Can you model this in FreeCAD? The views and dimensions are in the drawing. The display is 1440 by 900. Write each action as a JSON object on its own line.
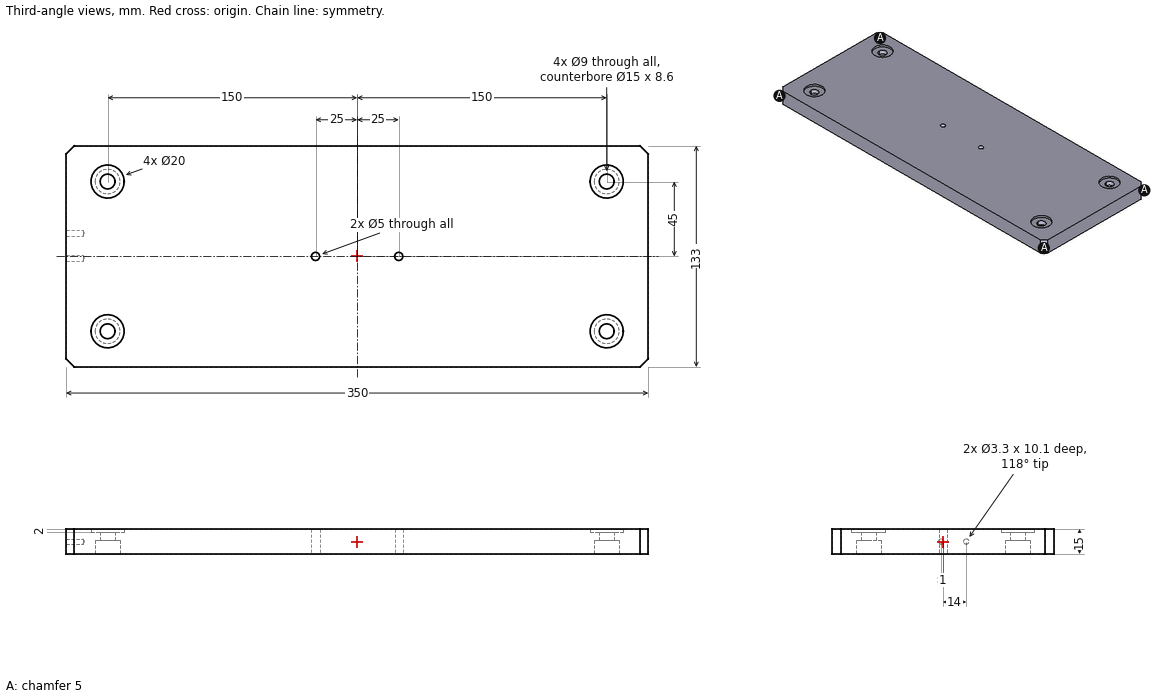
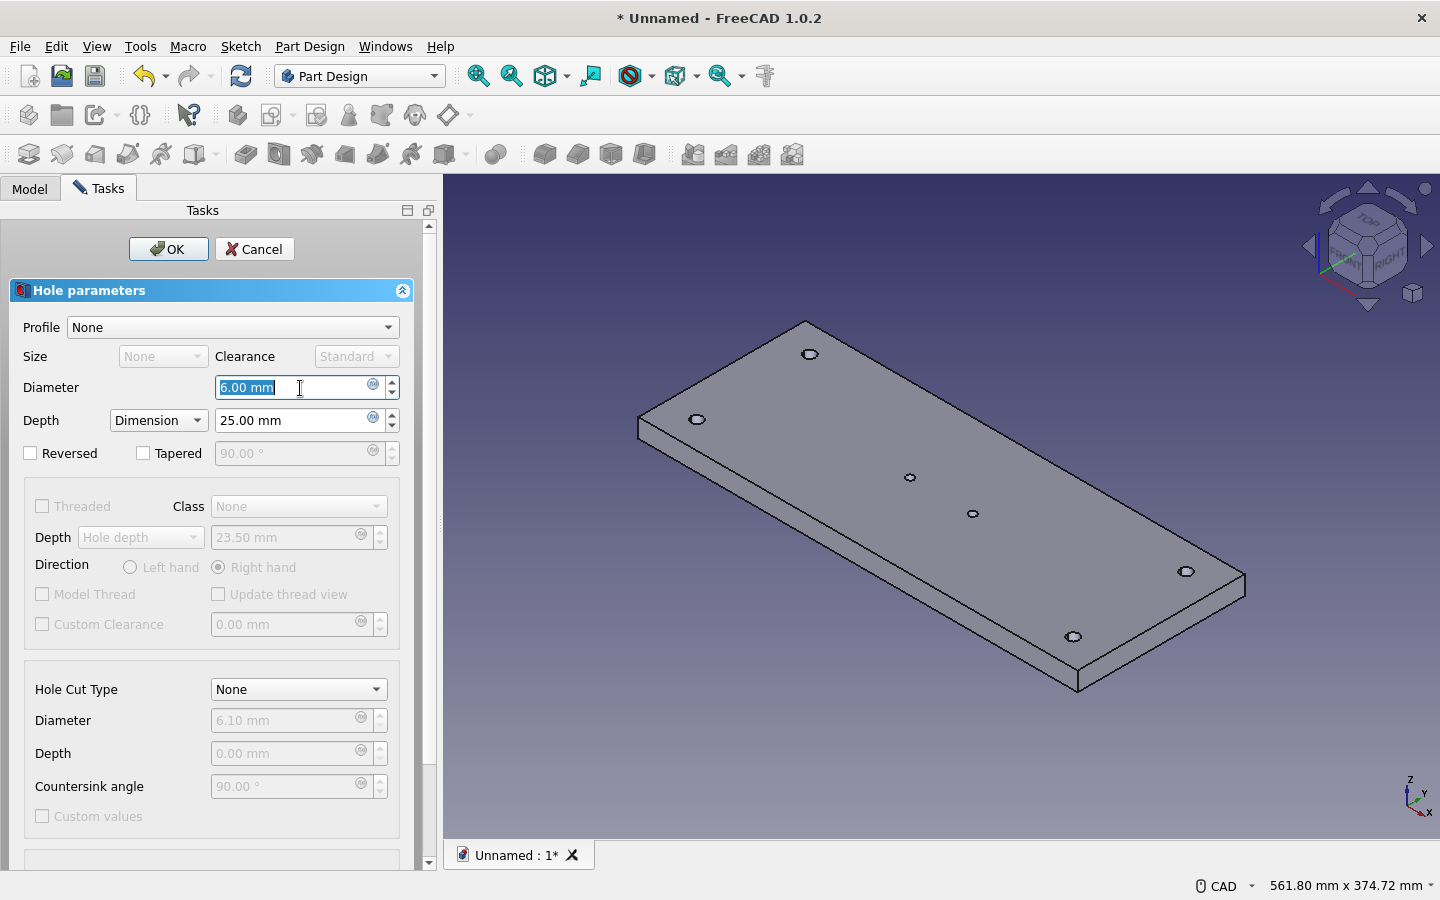
{"action": "type", "text": "5"}
{"action": "key", "text": "Tab"}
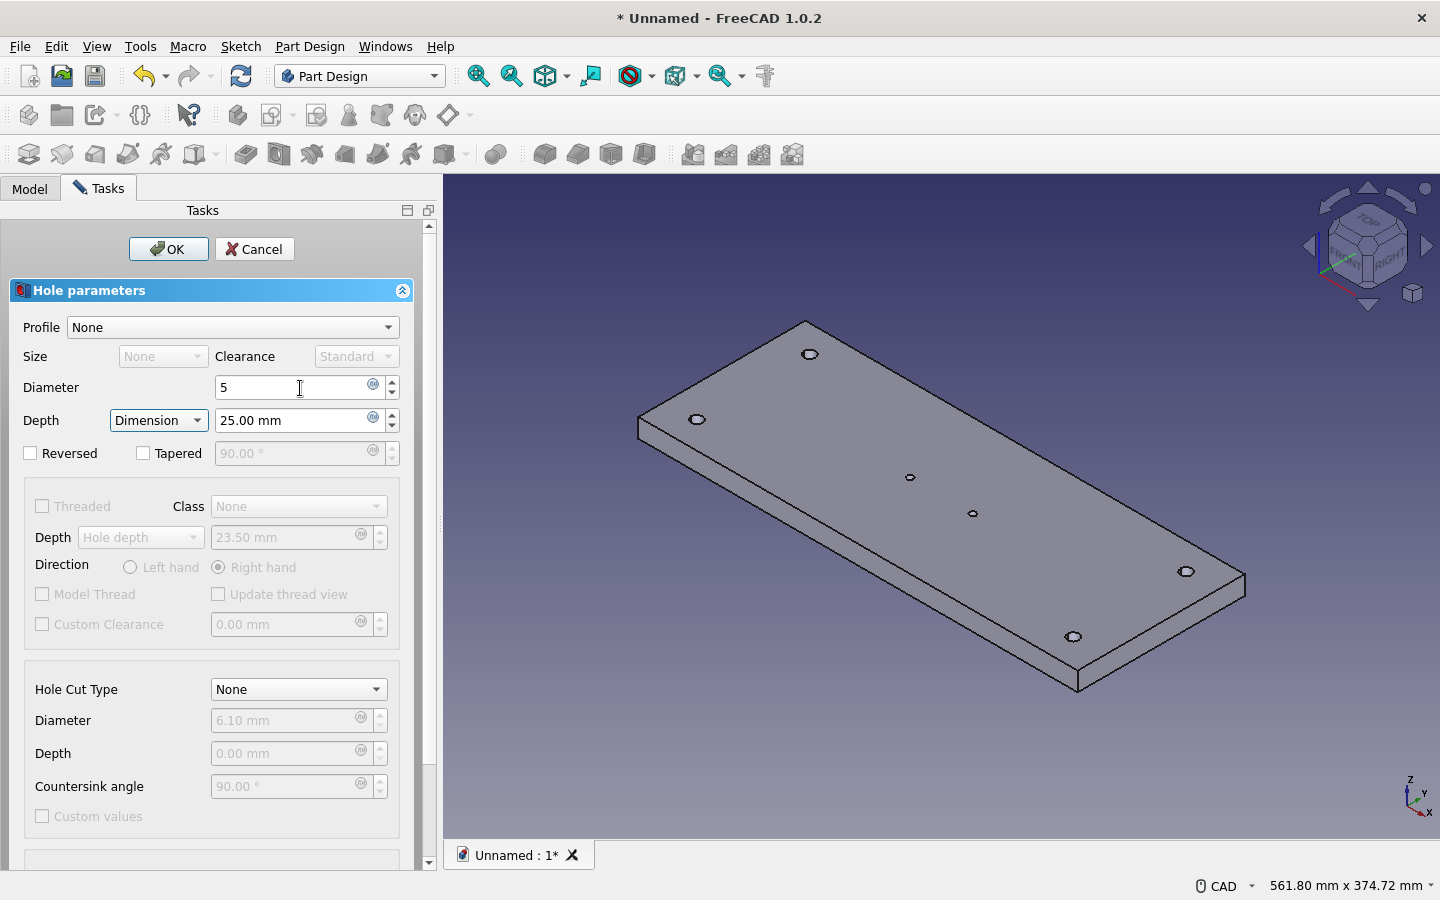
{"action": "left_click", "coordinate": [160, 420]}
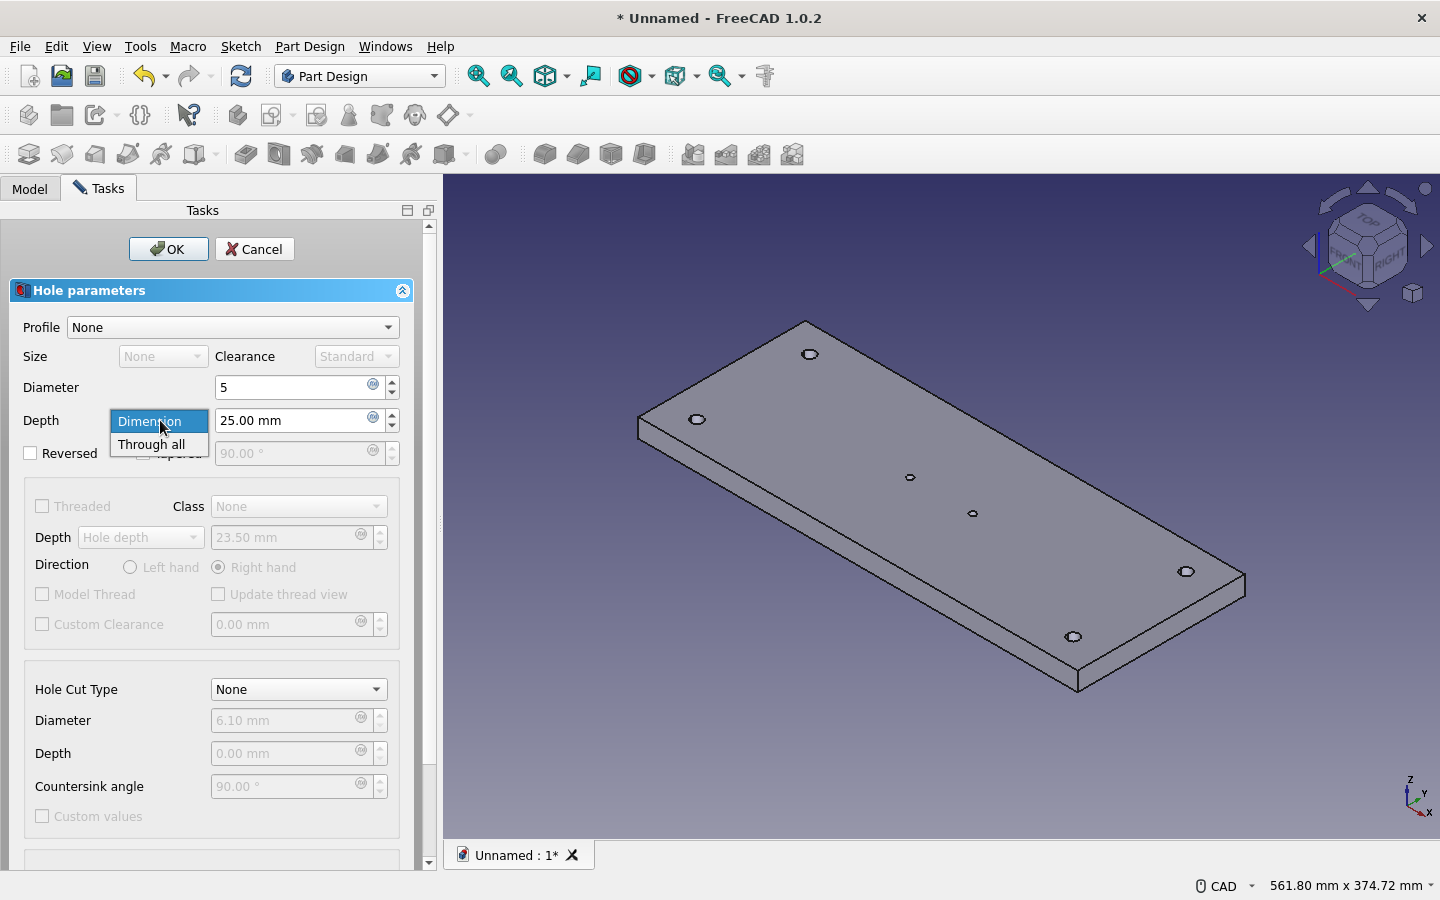
{"action": "left_click", "coordinate": [158, 444]}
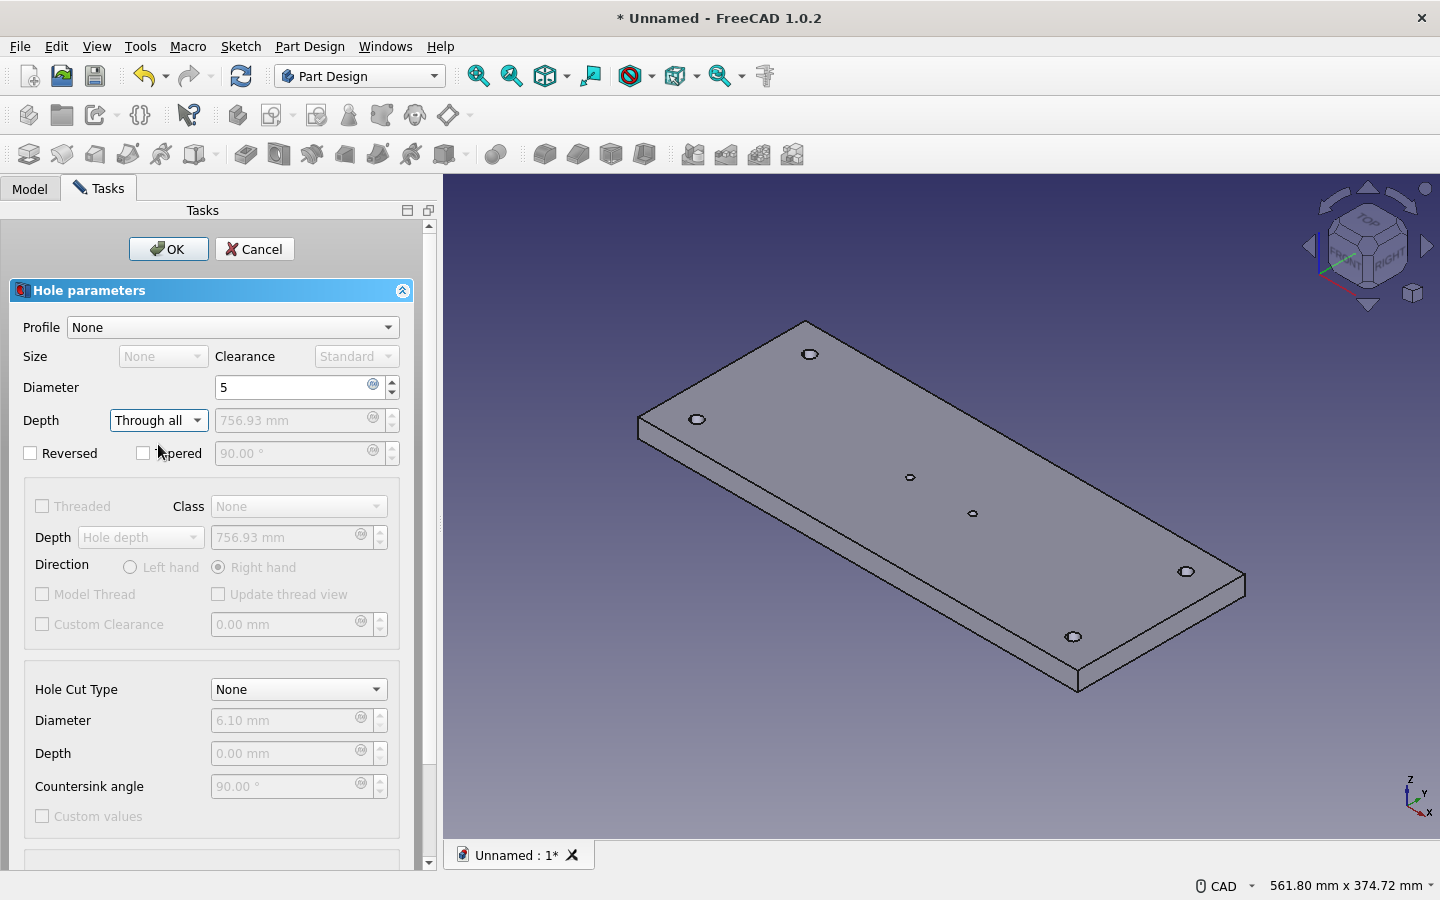
{"action": "left_click", "coordinate": [169, 249]}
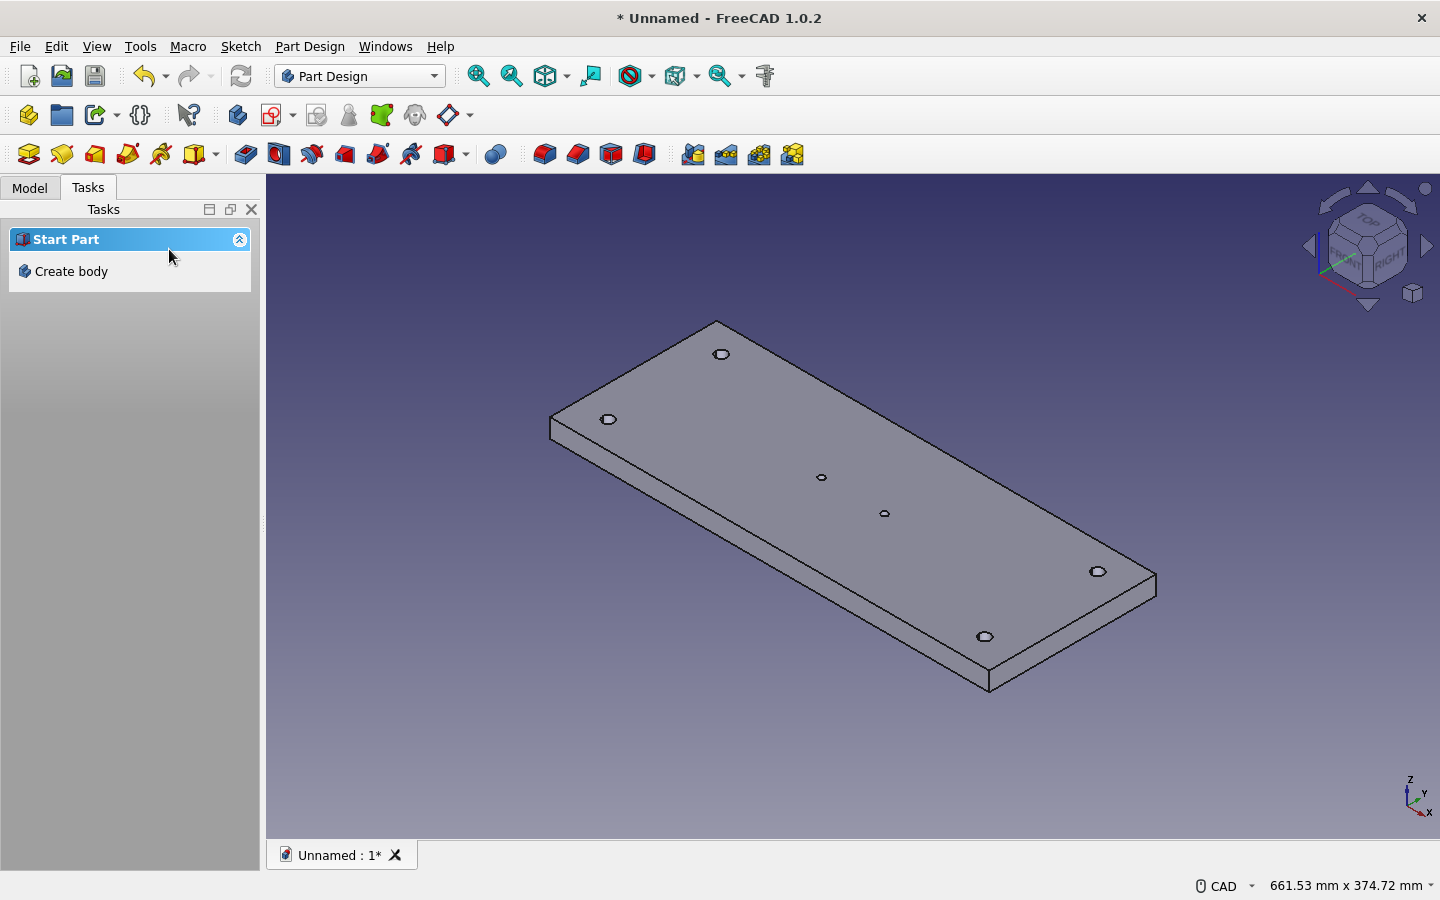
{"action": "left_click", "coordinate": [978, 567]}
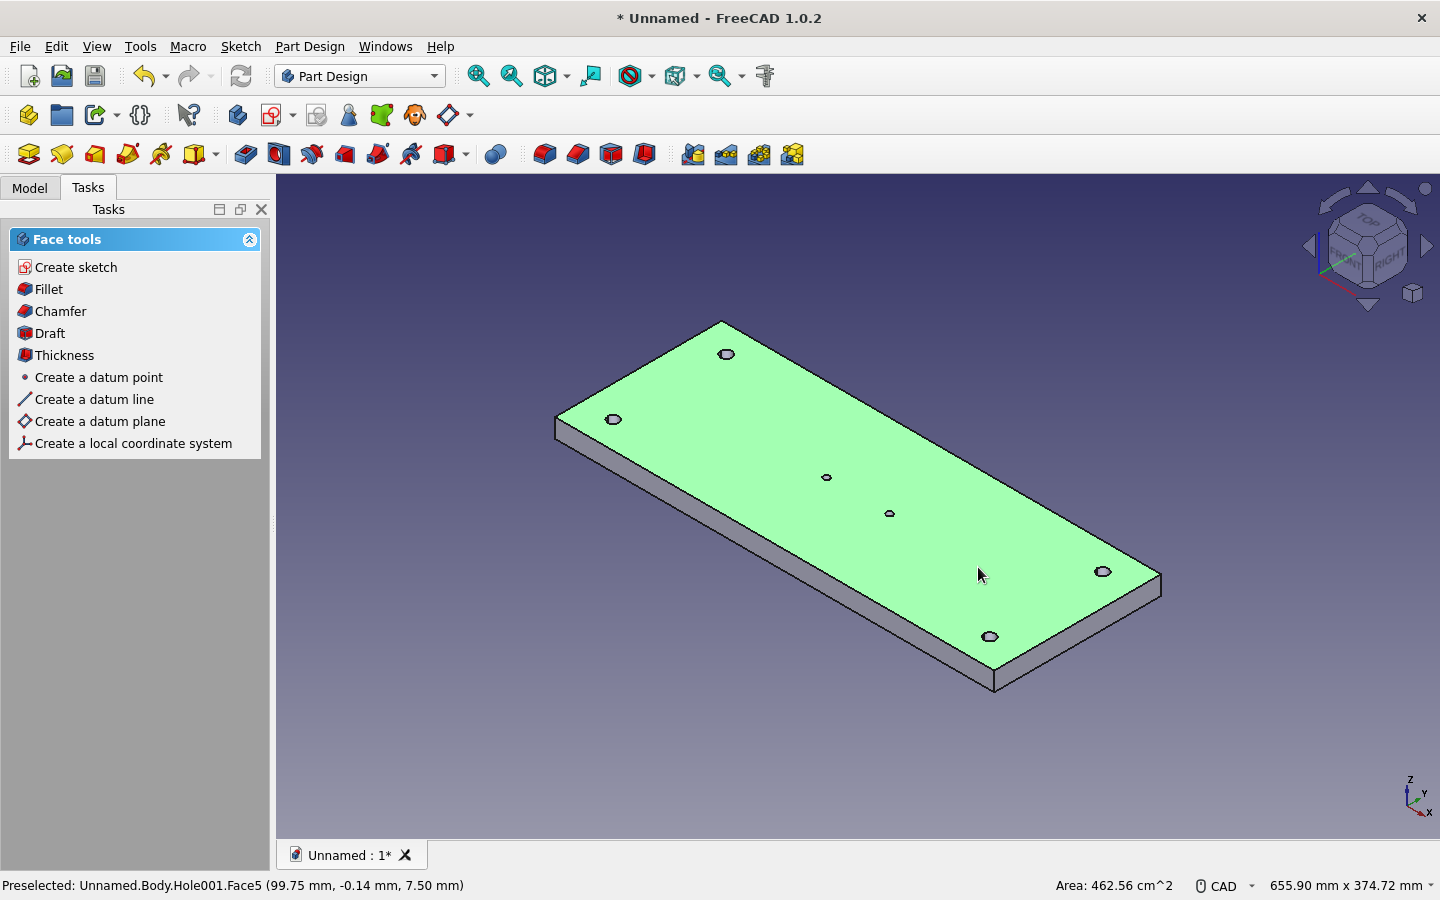
{"action": "left_click", "coordinate": [270, 116]}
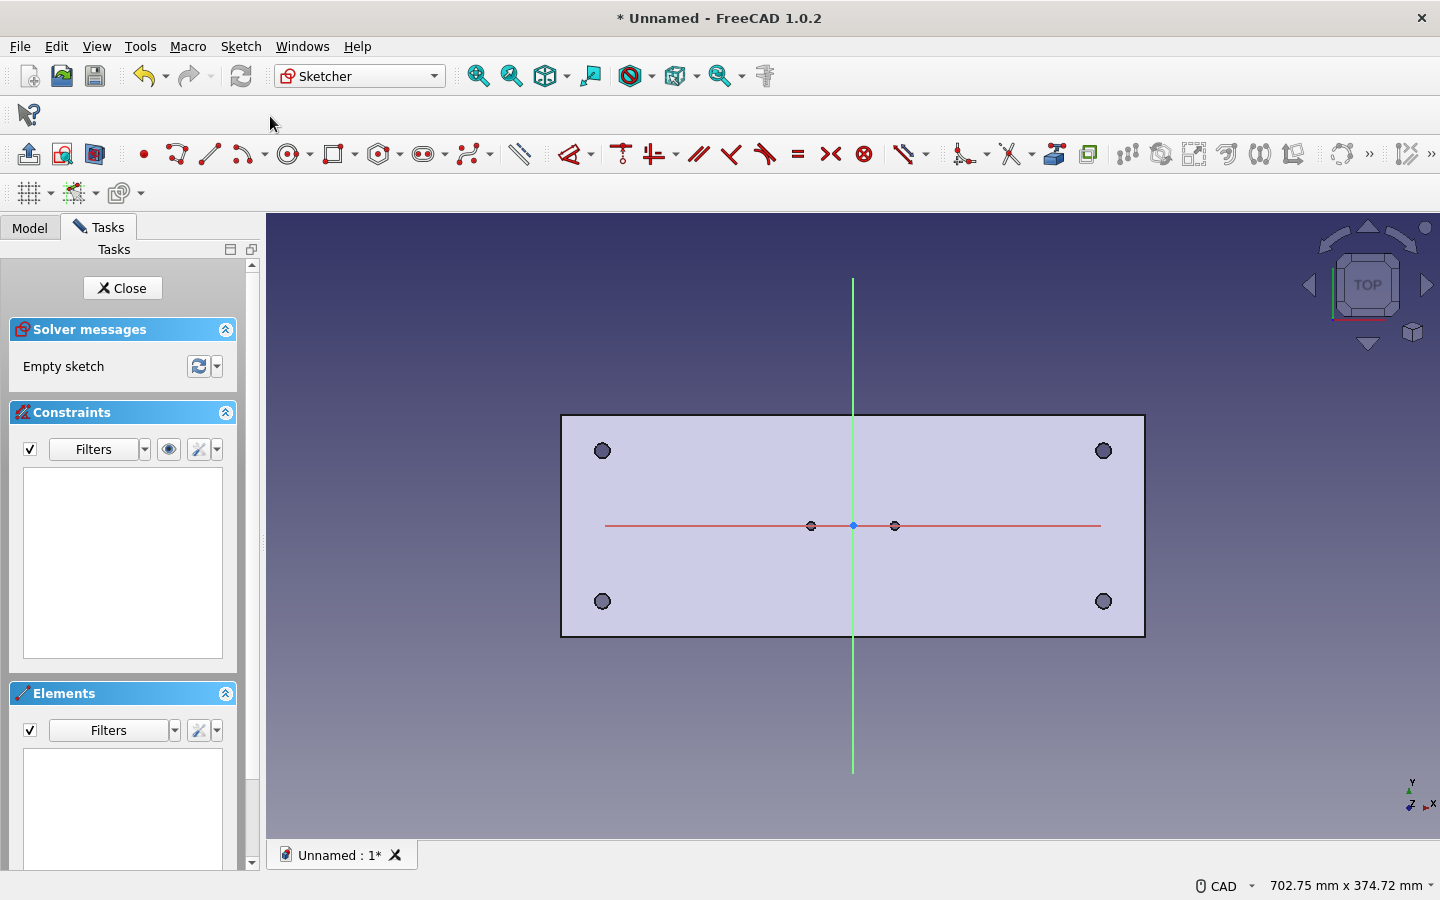
{"action": "key", "text": "g c"}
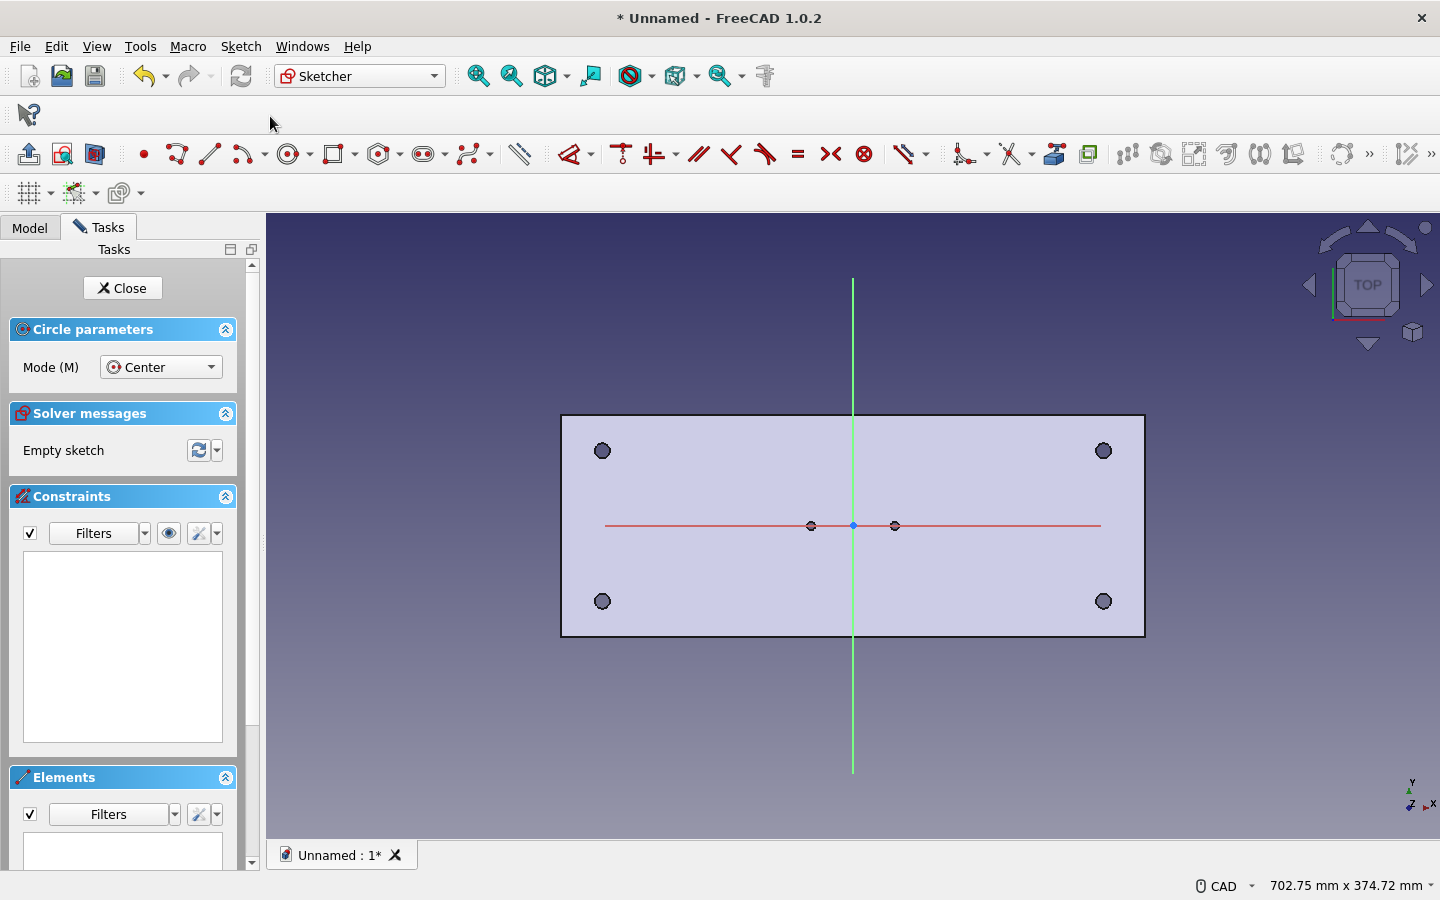
{"action": "scroll", "coordinate": [602, 451], "scroll_direction": "up", "scroll_amount": 2}